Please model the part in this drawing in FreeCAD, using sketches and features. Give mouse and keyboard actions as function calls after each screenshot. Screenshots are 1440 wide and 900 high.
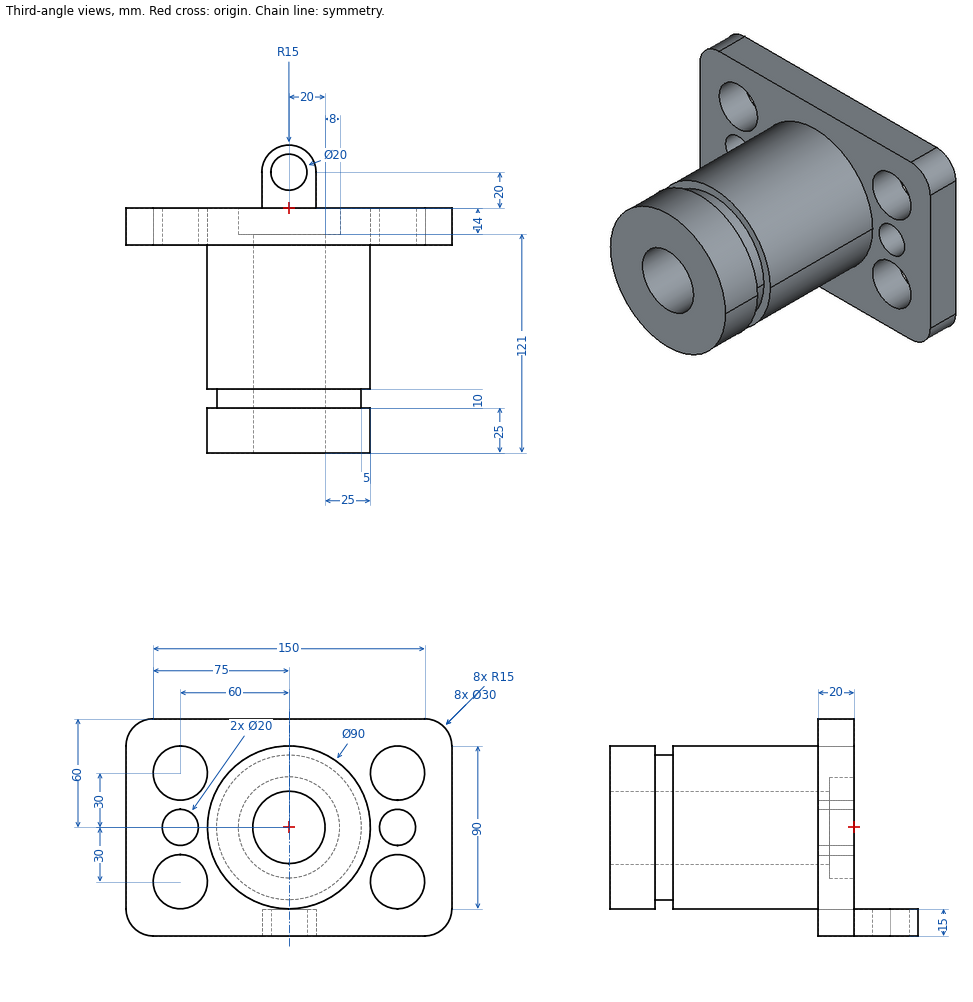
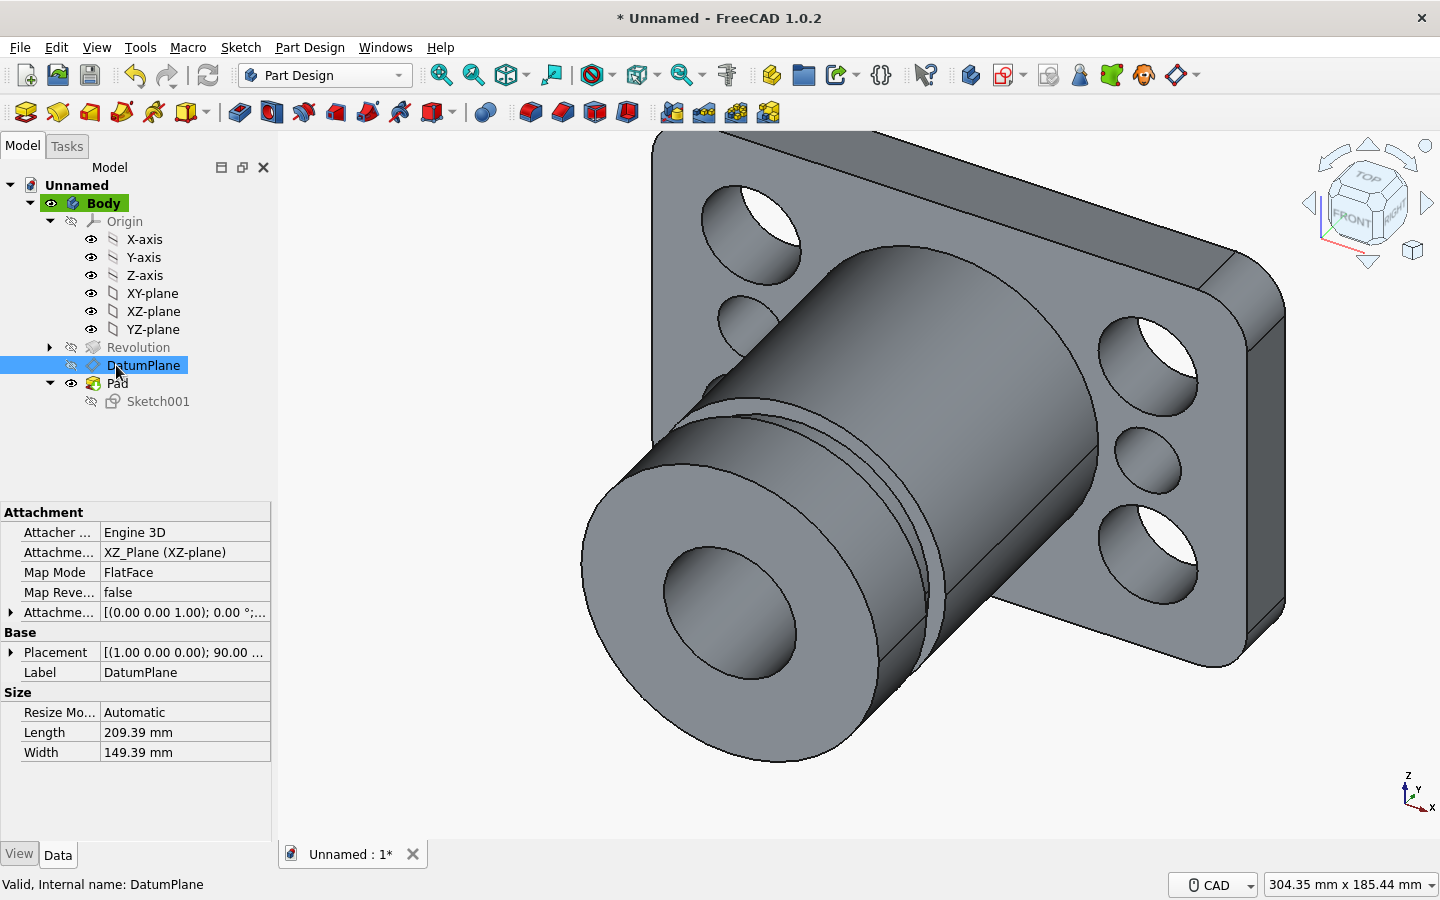
click(442, 76)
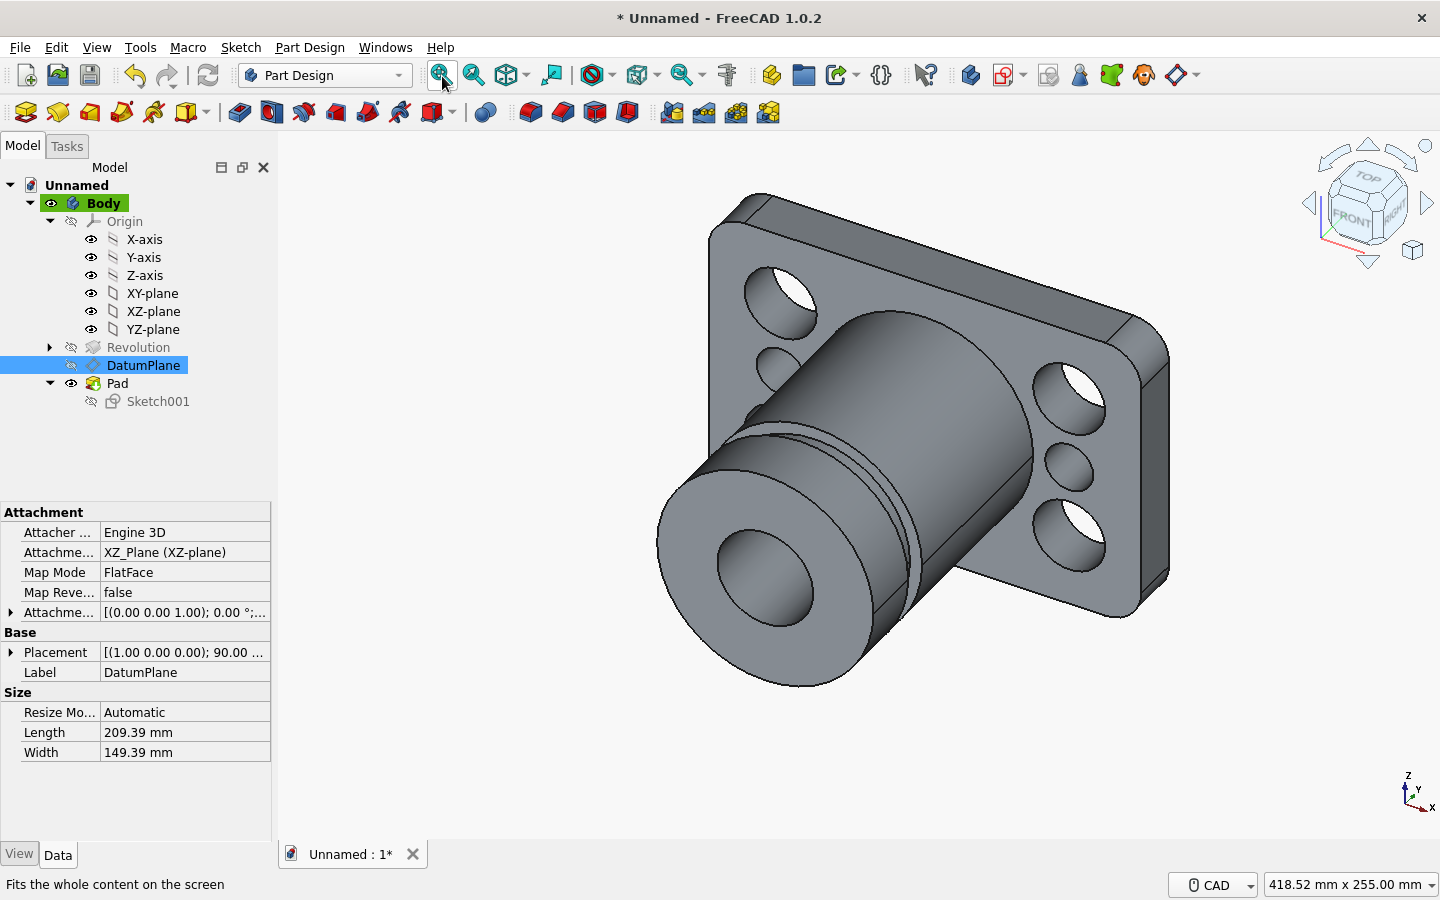
key(5)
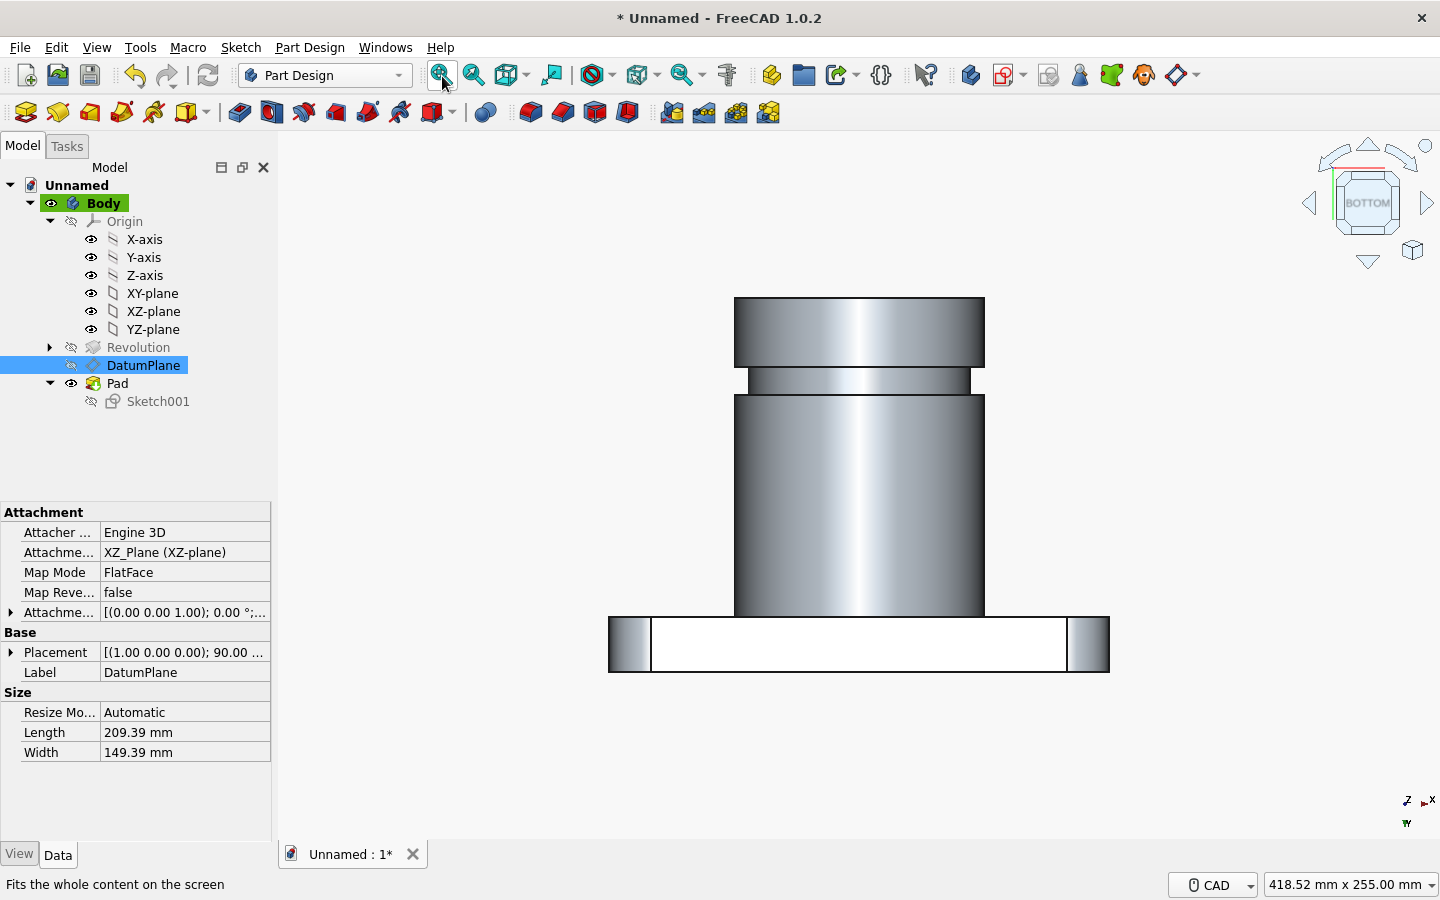
click(1037, 644)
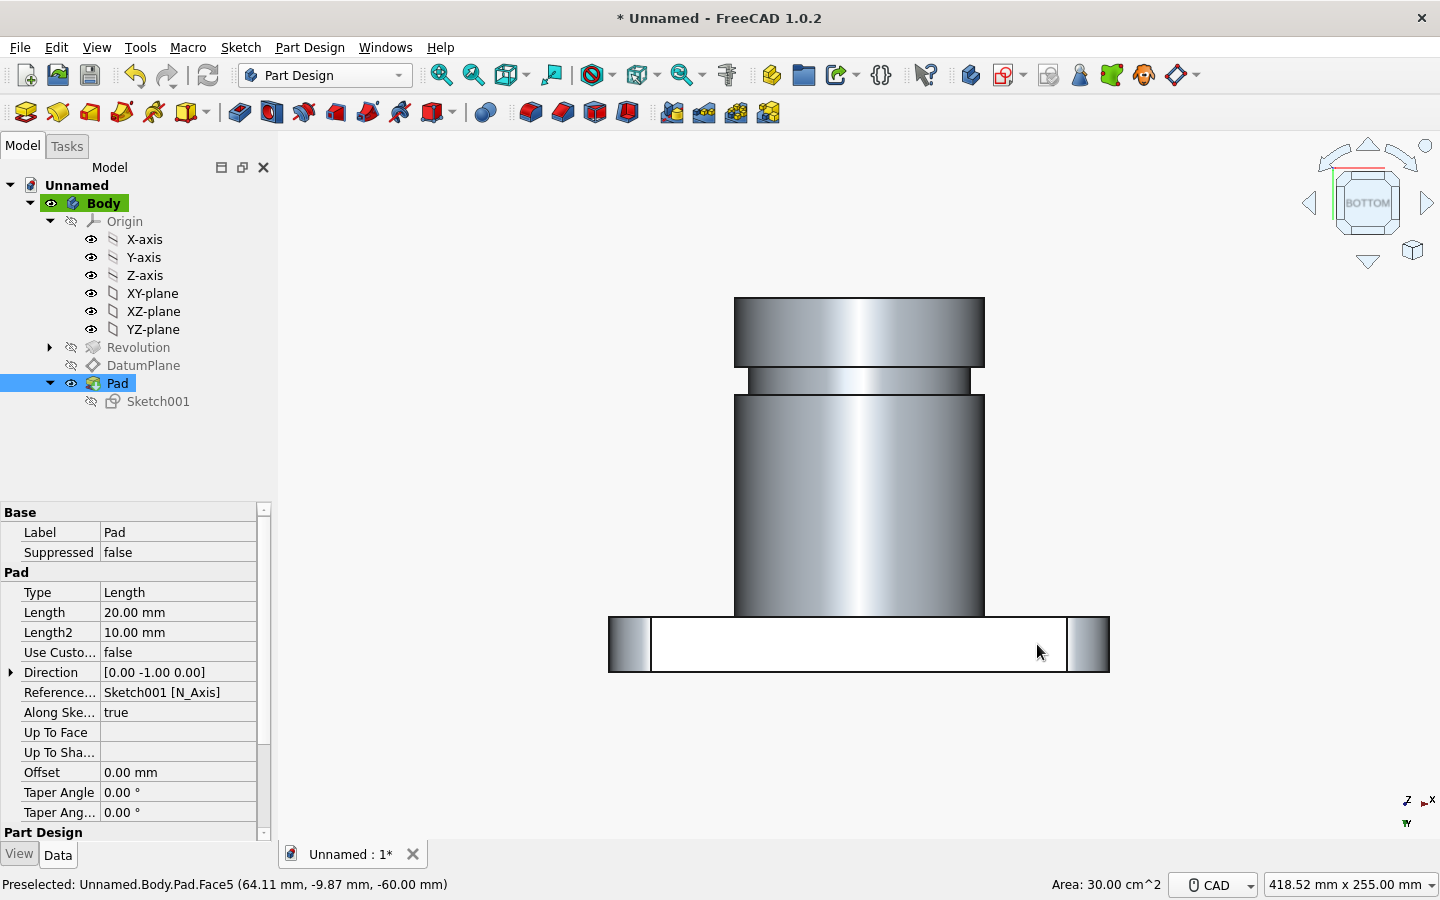
click(1004, 76)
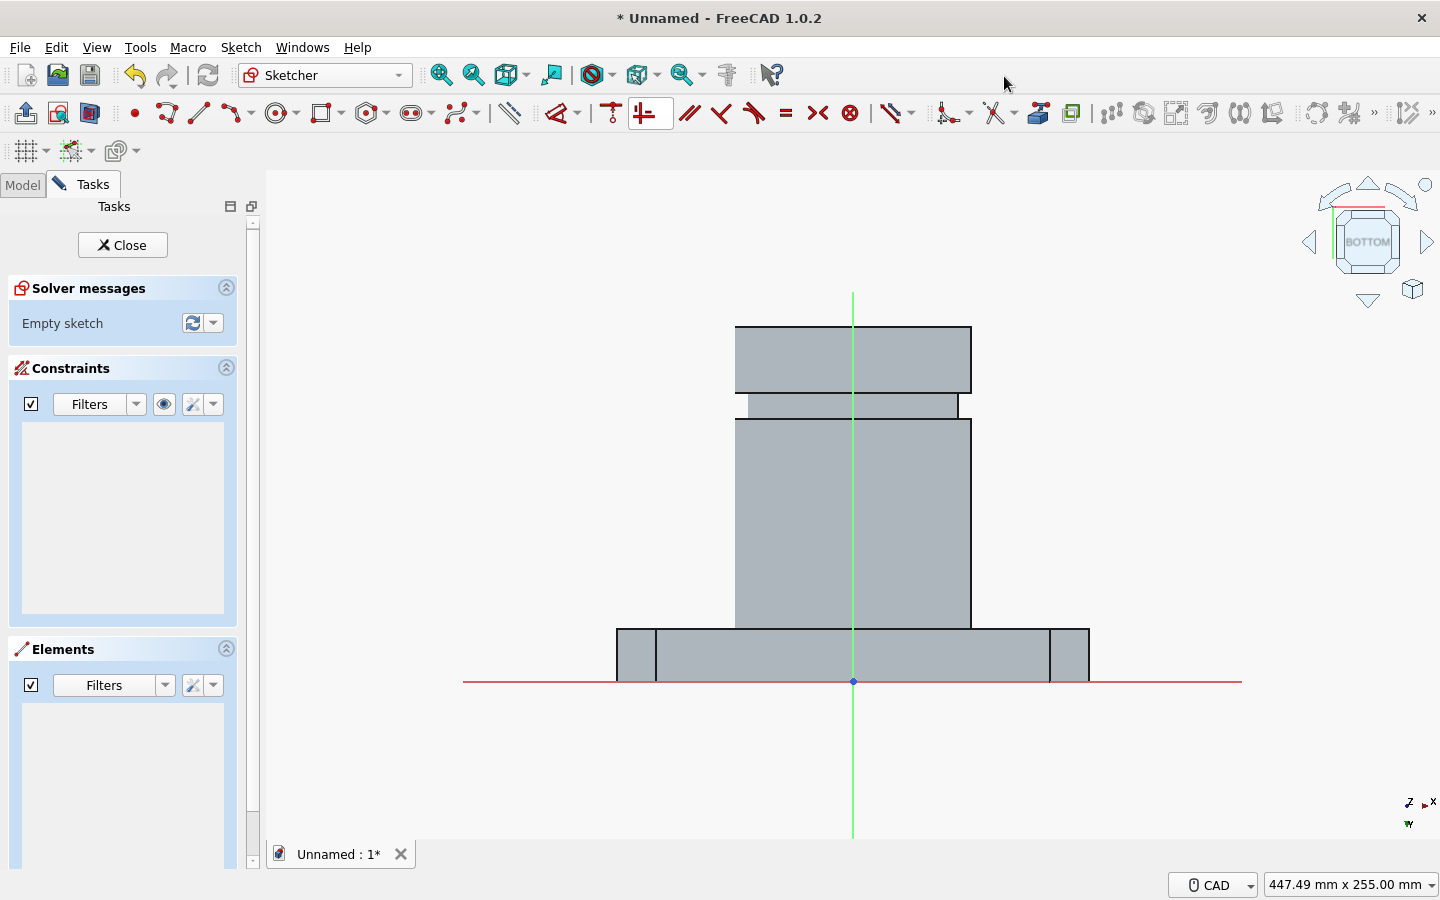
scroll(870, 784, up, 8)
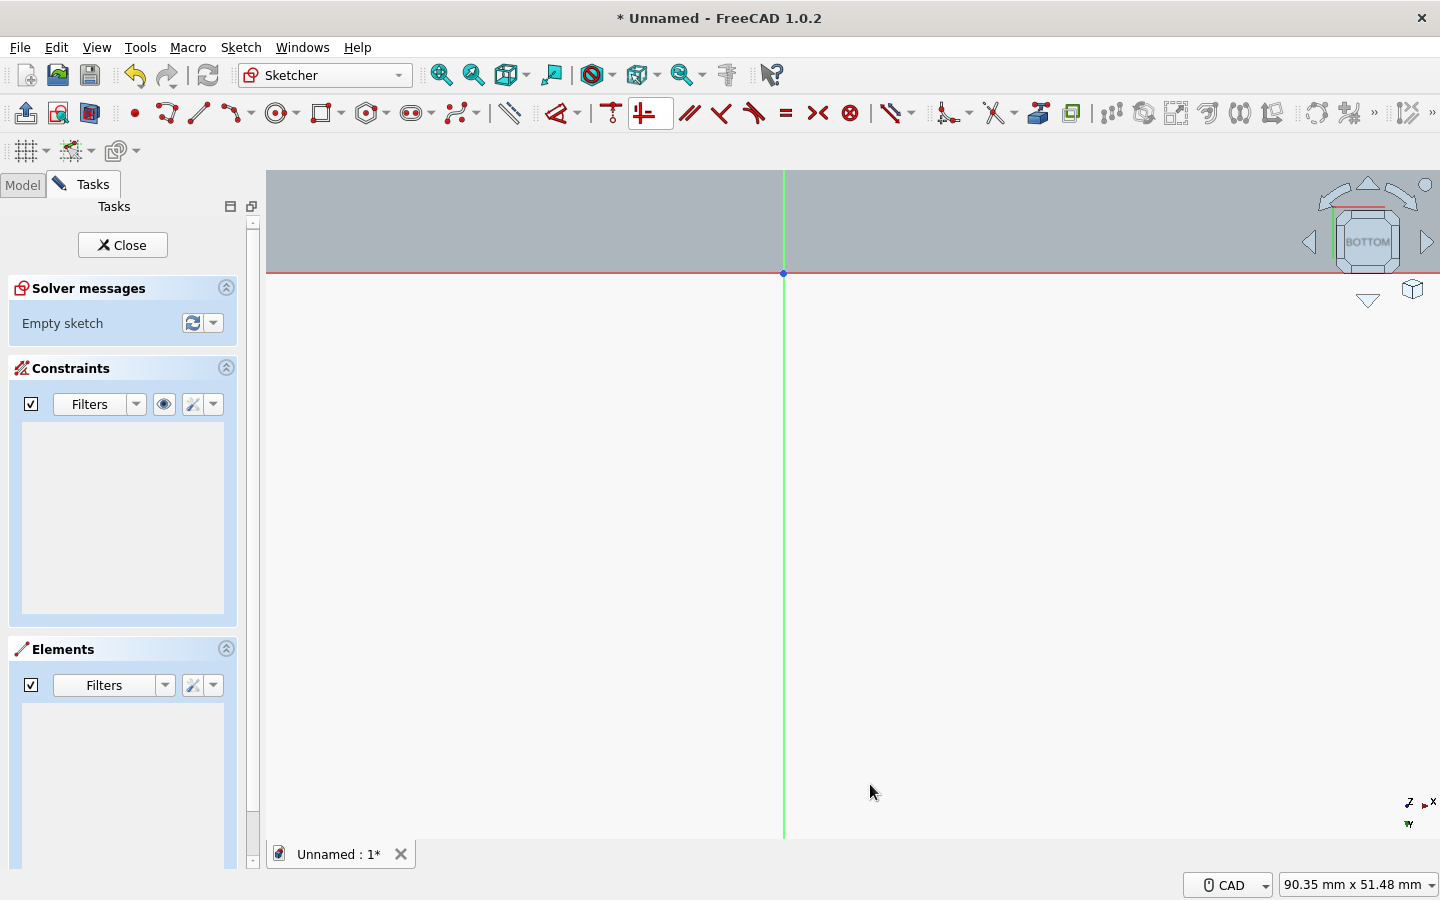
click(168, 114)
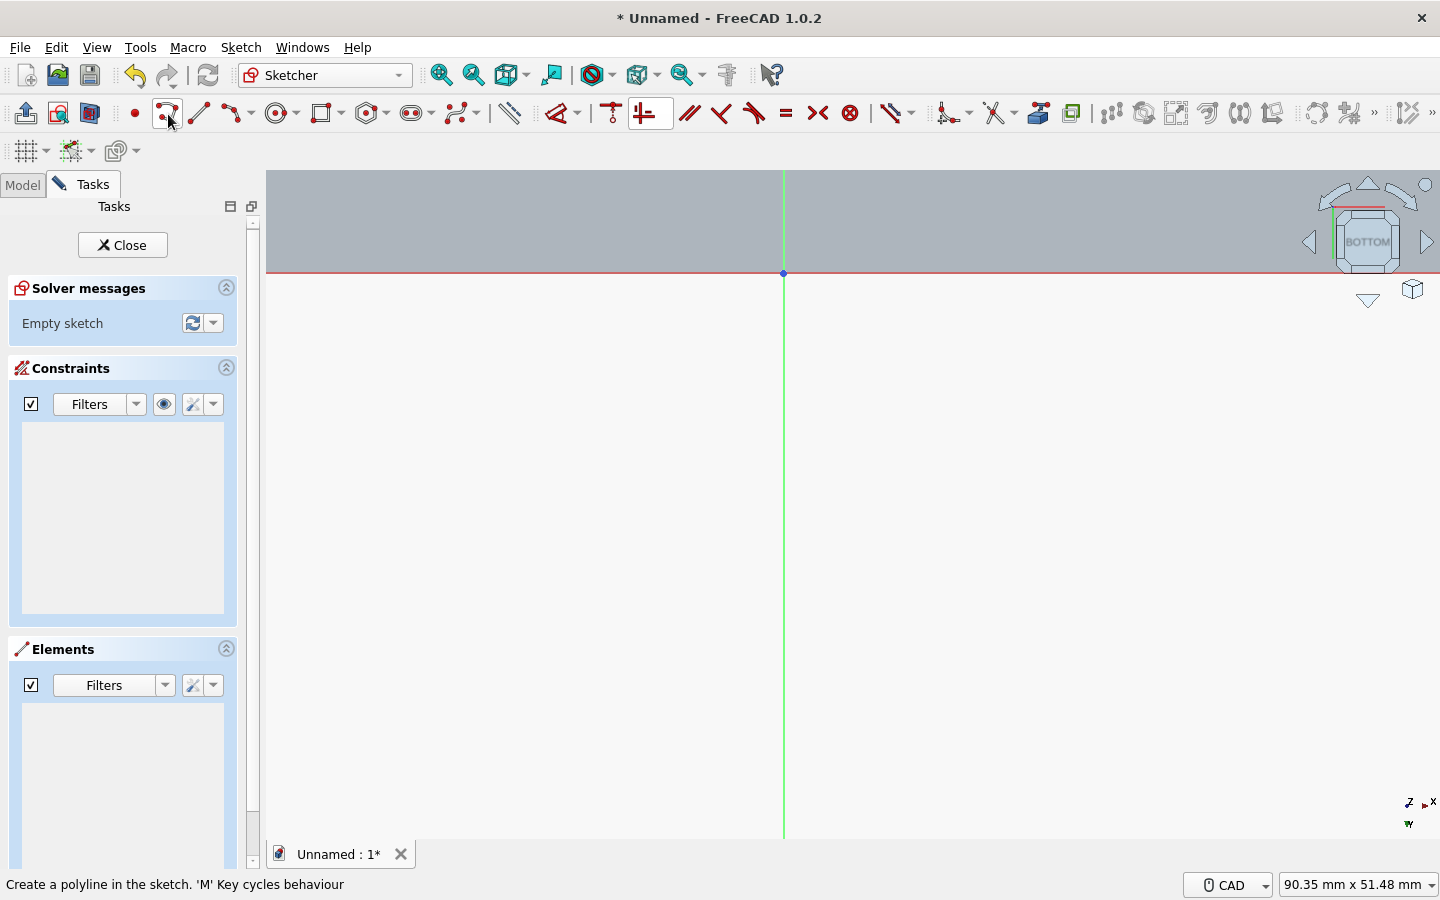
click(979, 533)
click(979, 273)
click(589, 282)
click(589, 533)
right_click(589, 533)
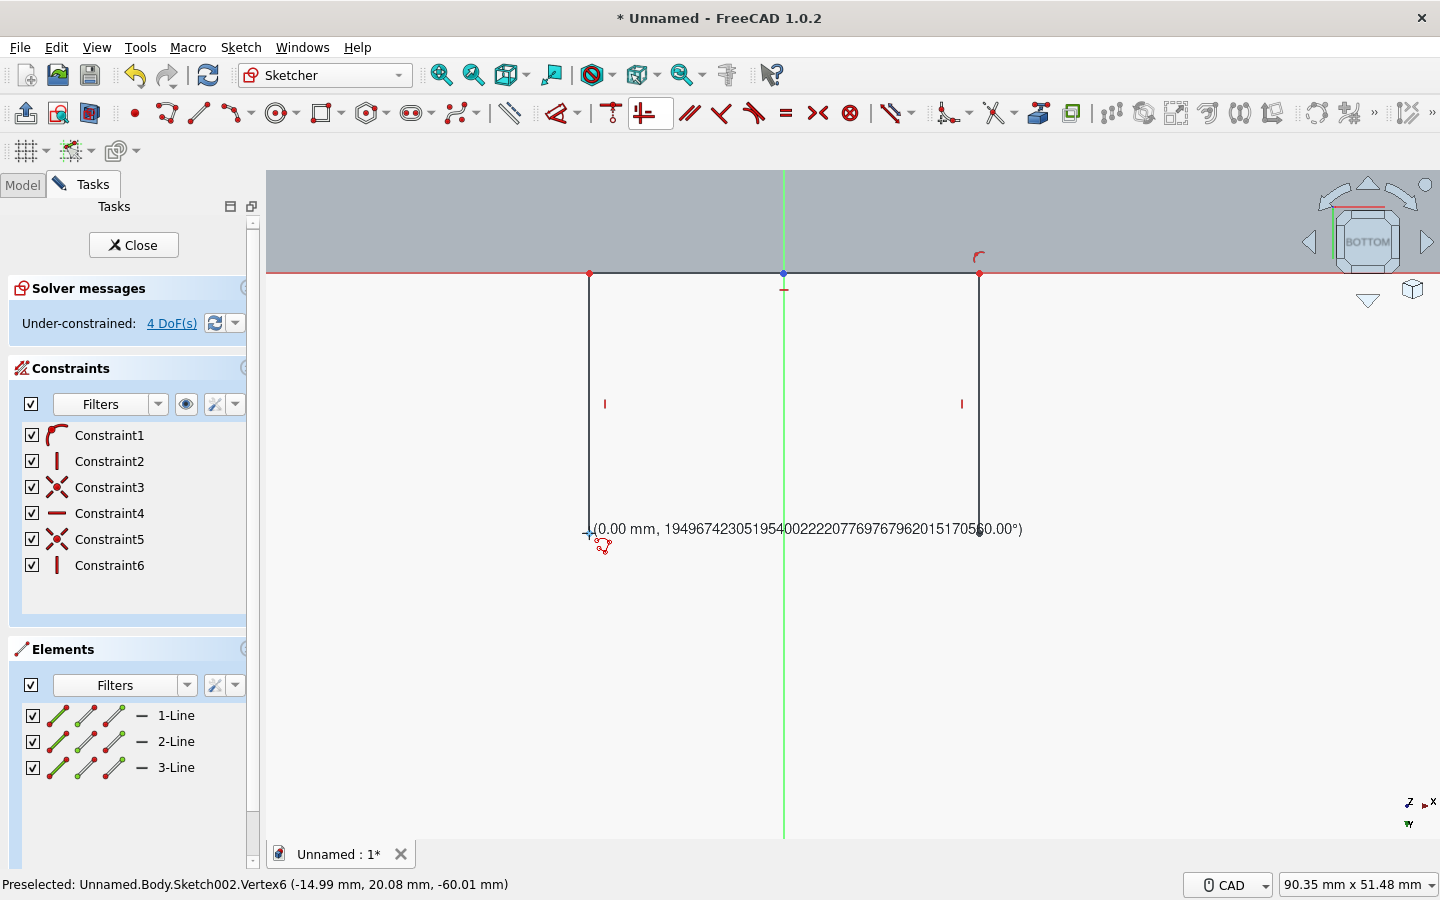
click(232, 114)